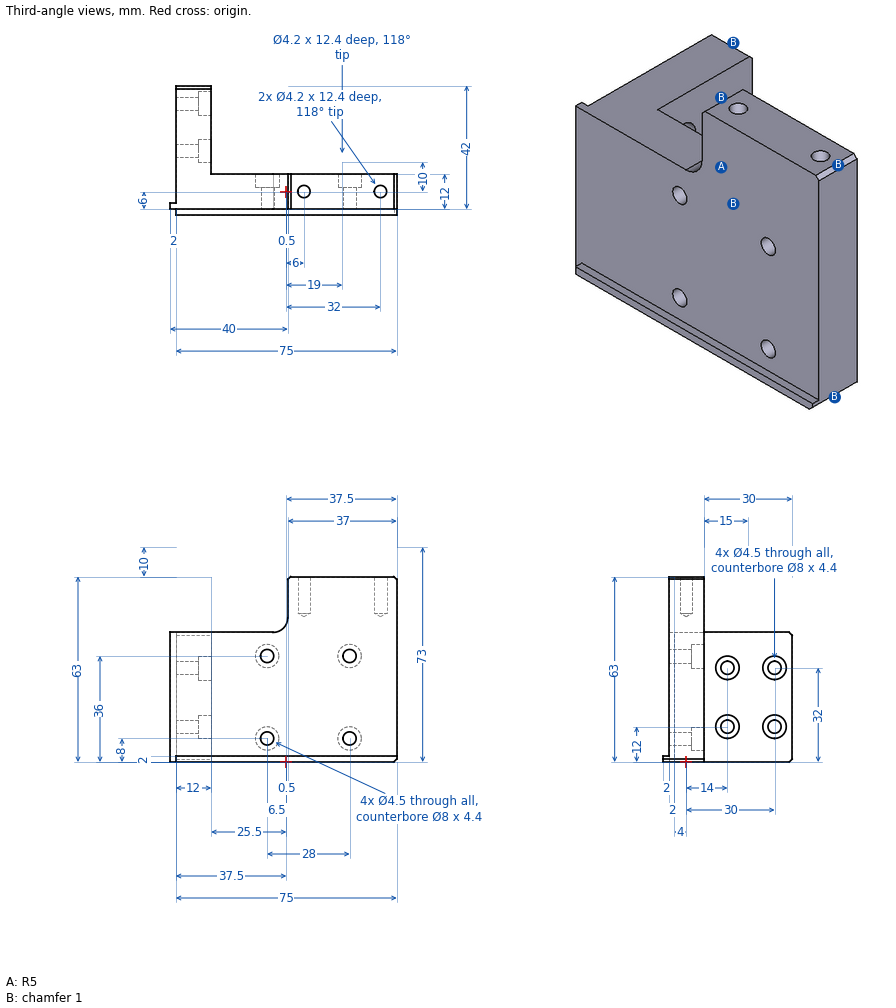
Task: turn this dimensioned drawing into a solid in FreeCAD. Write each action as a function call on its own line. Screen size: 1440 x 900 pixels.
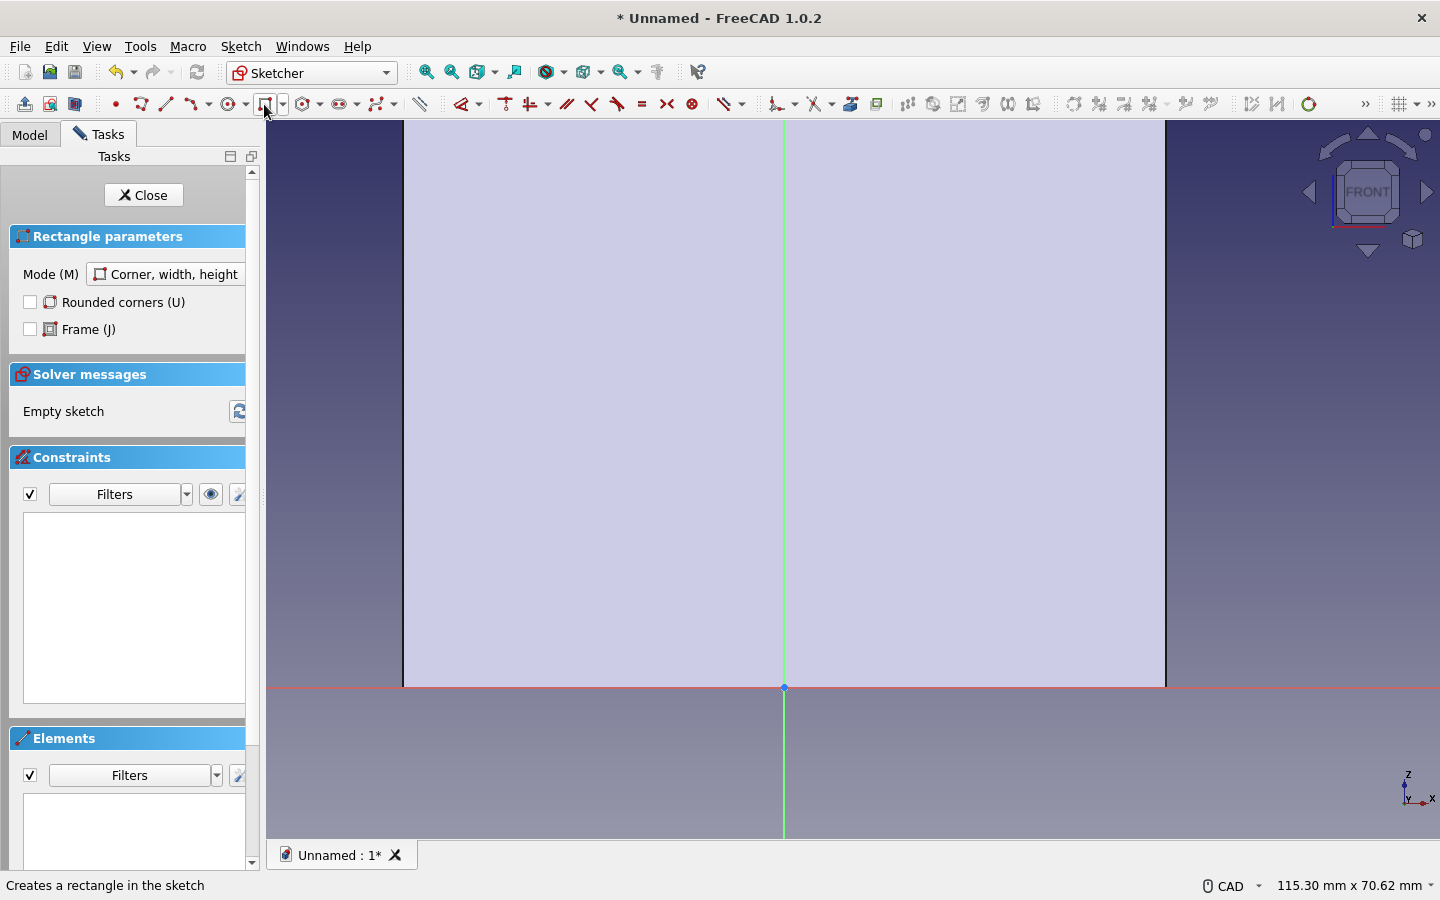
click(403, 667)
click(1166, 688)
key(Escape)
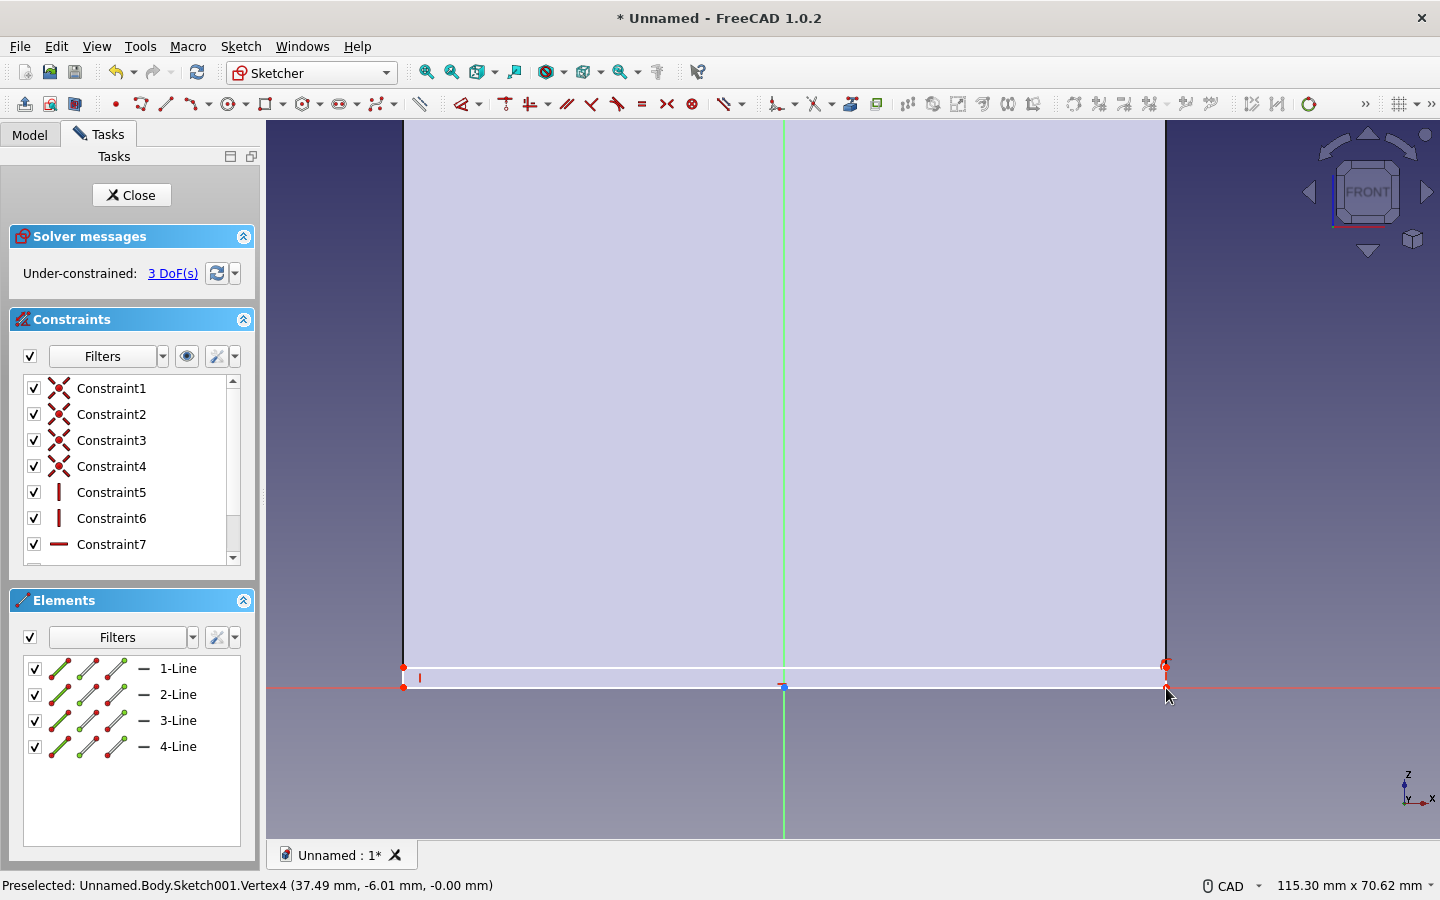
click(460, 104)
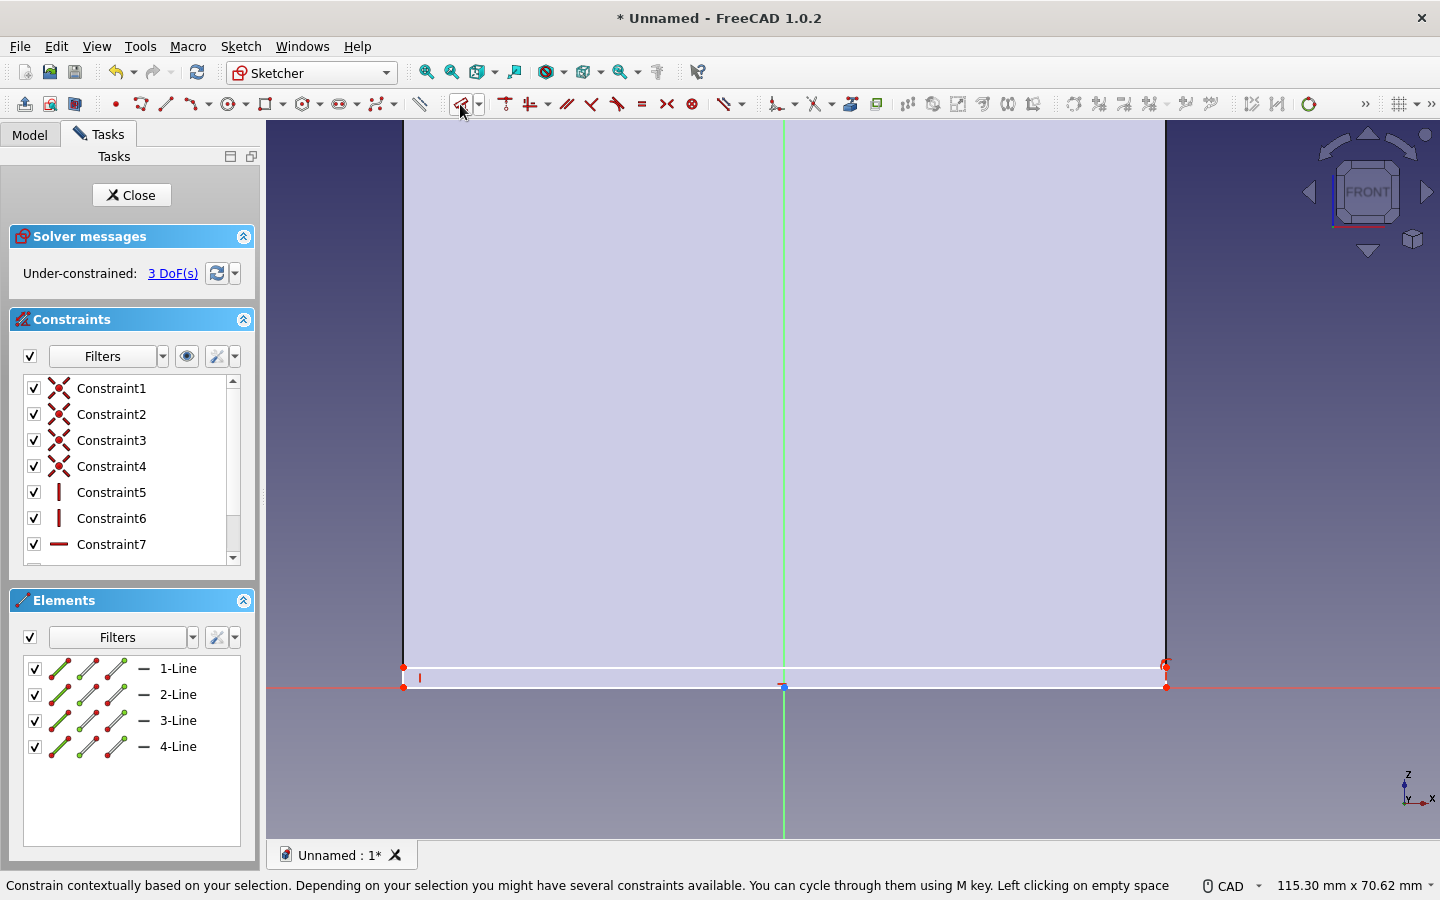
scroll(403, 678, up, 4)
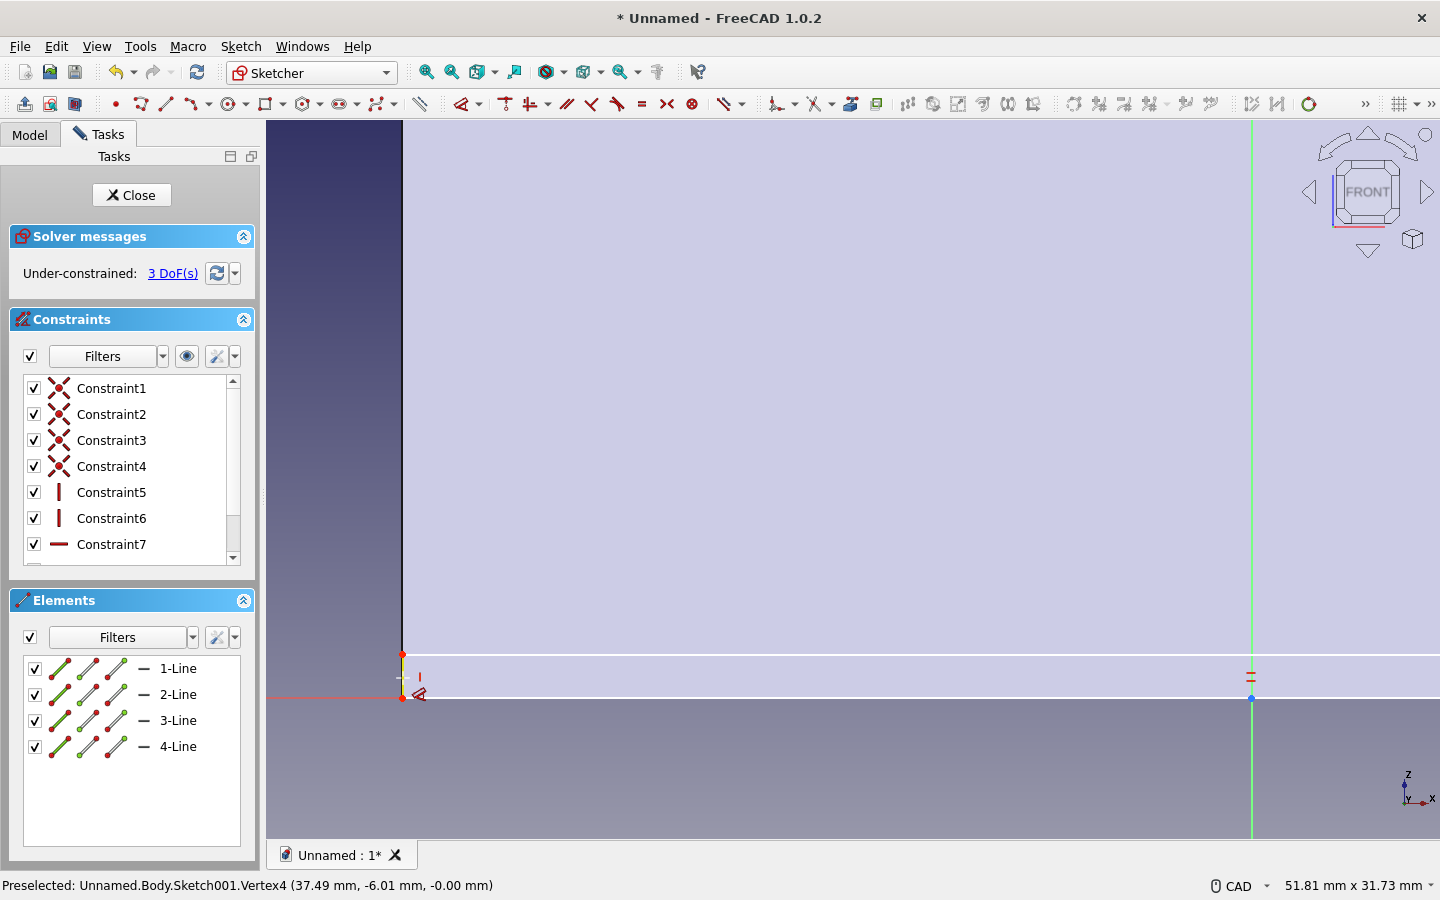
click(403, 677)
click(369, 677)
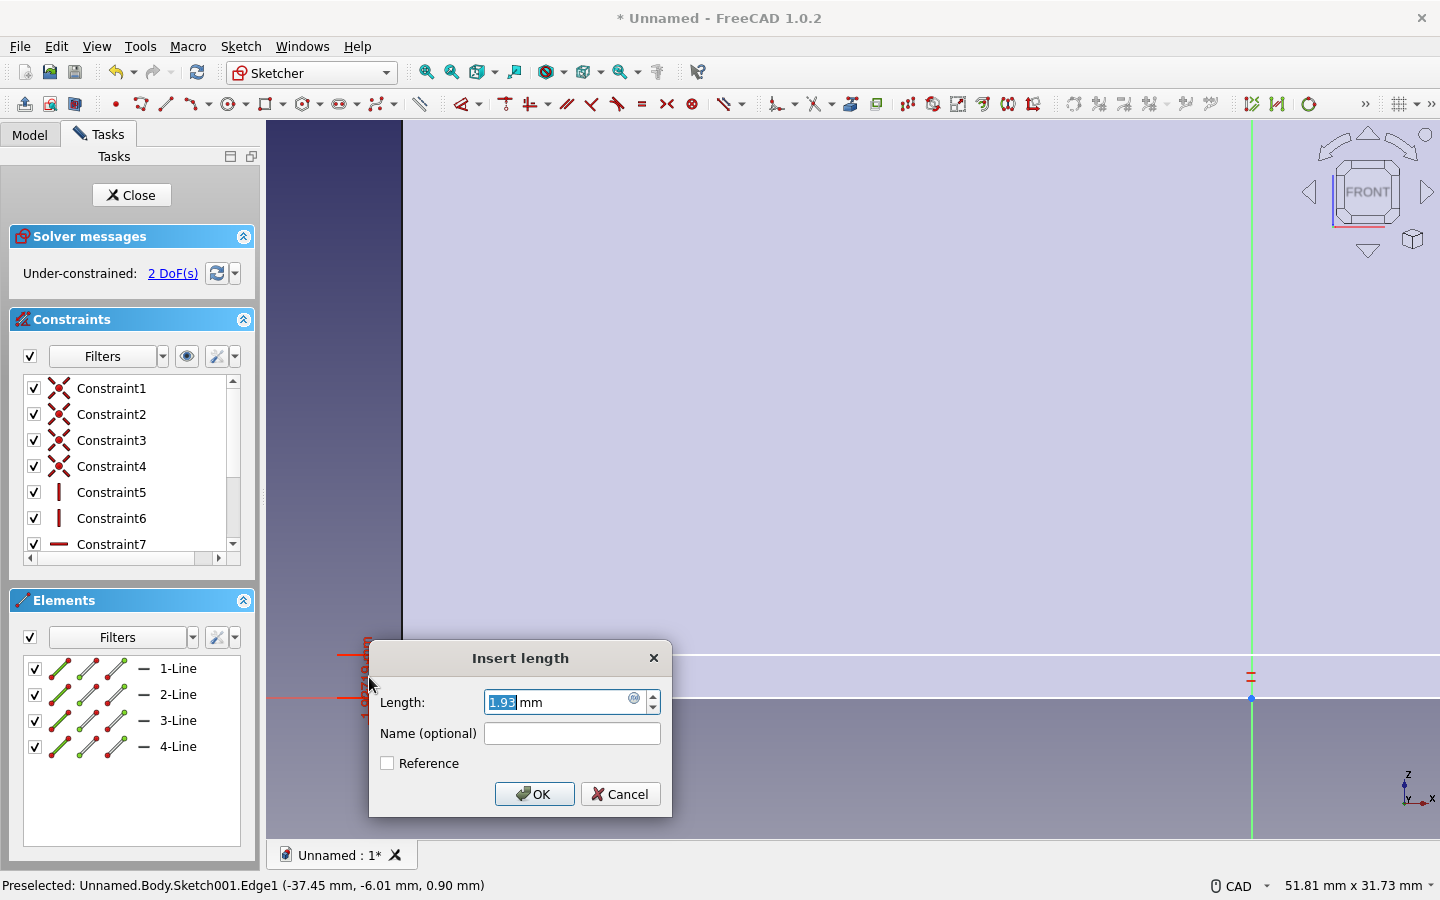
text(2)
key(Return)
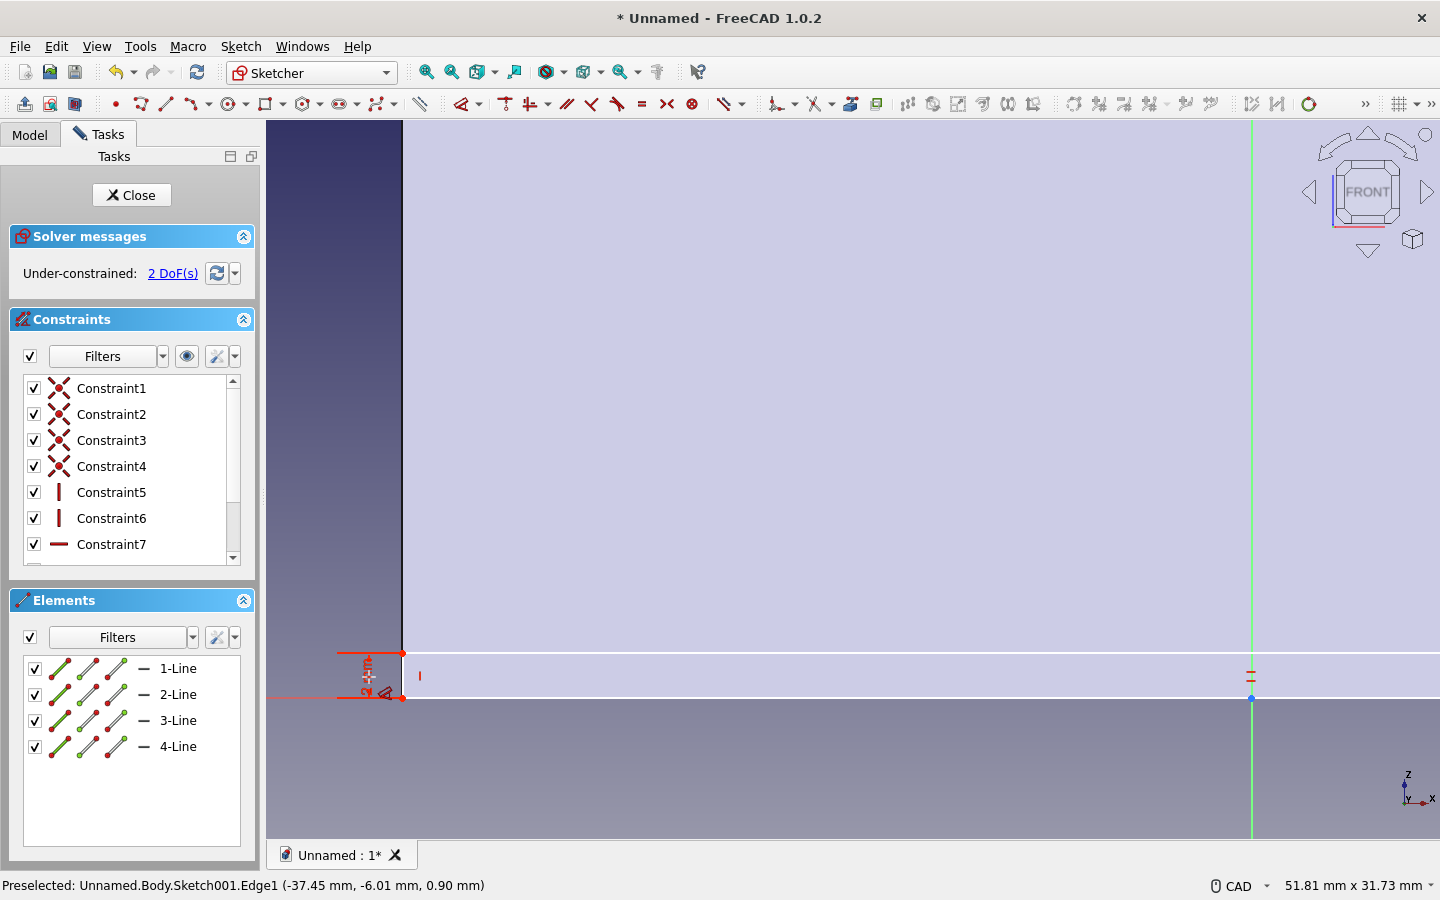
click(912, 698)
click(839, 732)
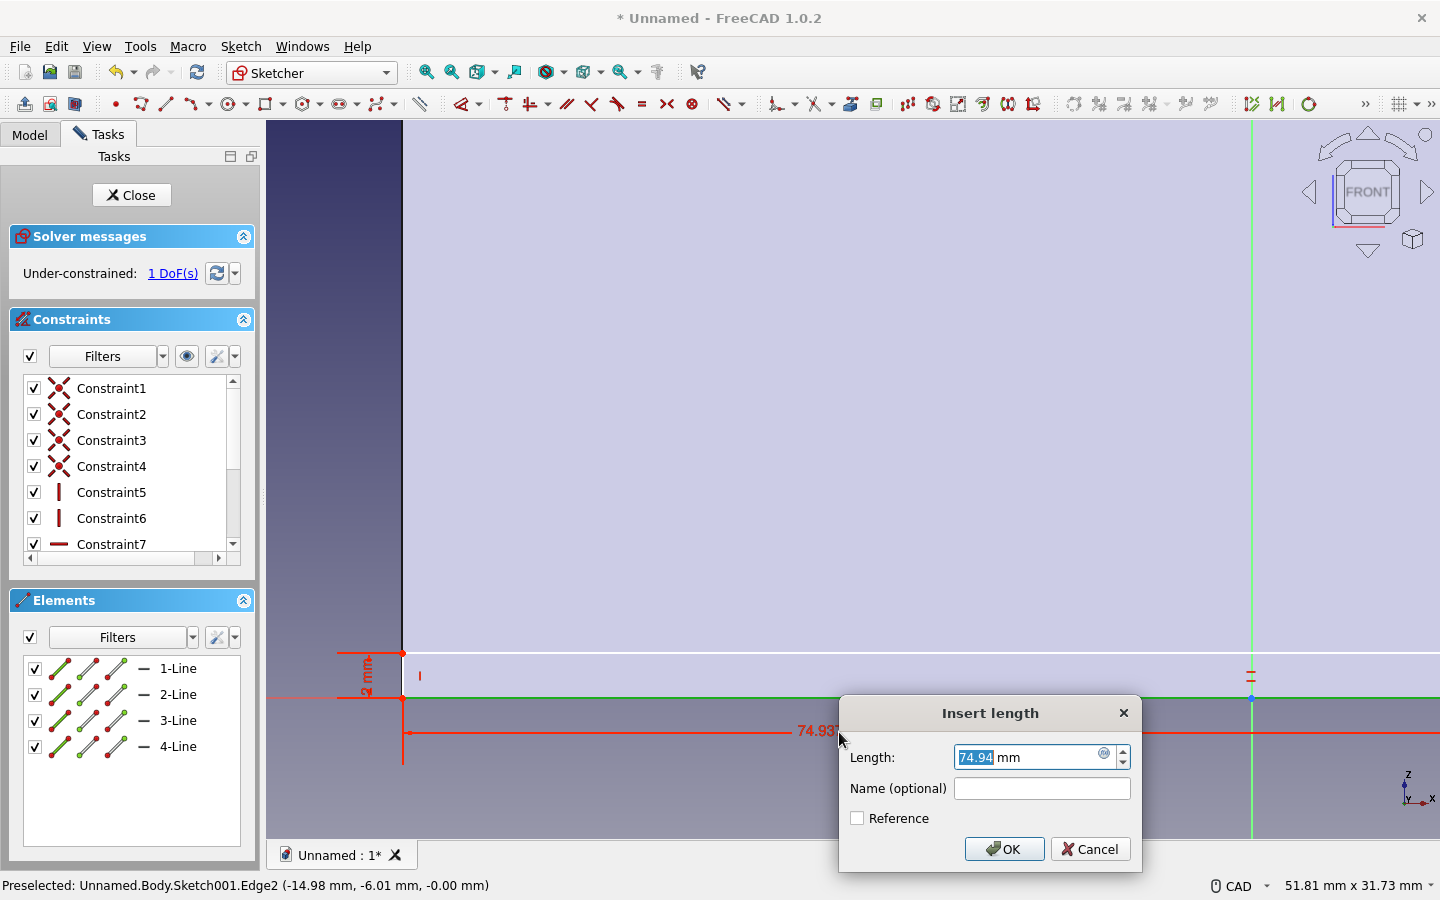
text(75)
key(Return)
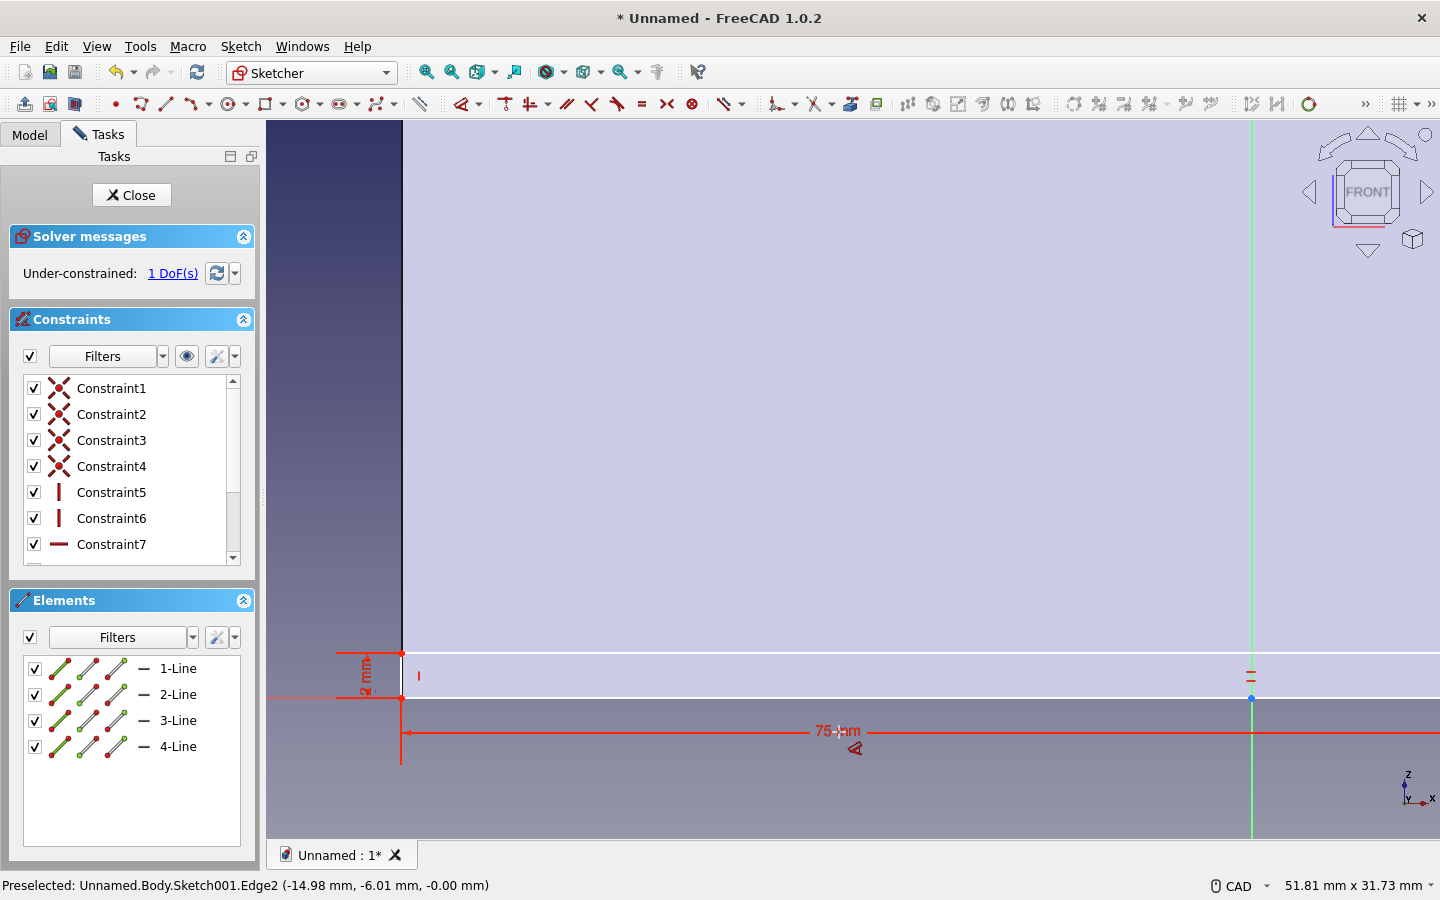
click(401, 653)
click(631, 732)